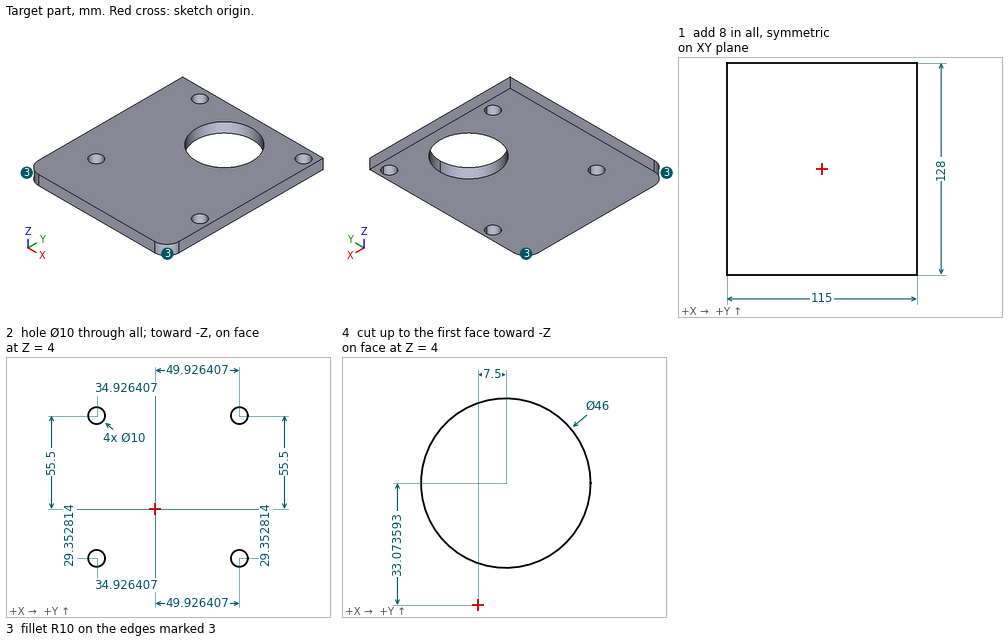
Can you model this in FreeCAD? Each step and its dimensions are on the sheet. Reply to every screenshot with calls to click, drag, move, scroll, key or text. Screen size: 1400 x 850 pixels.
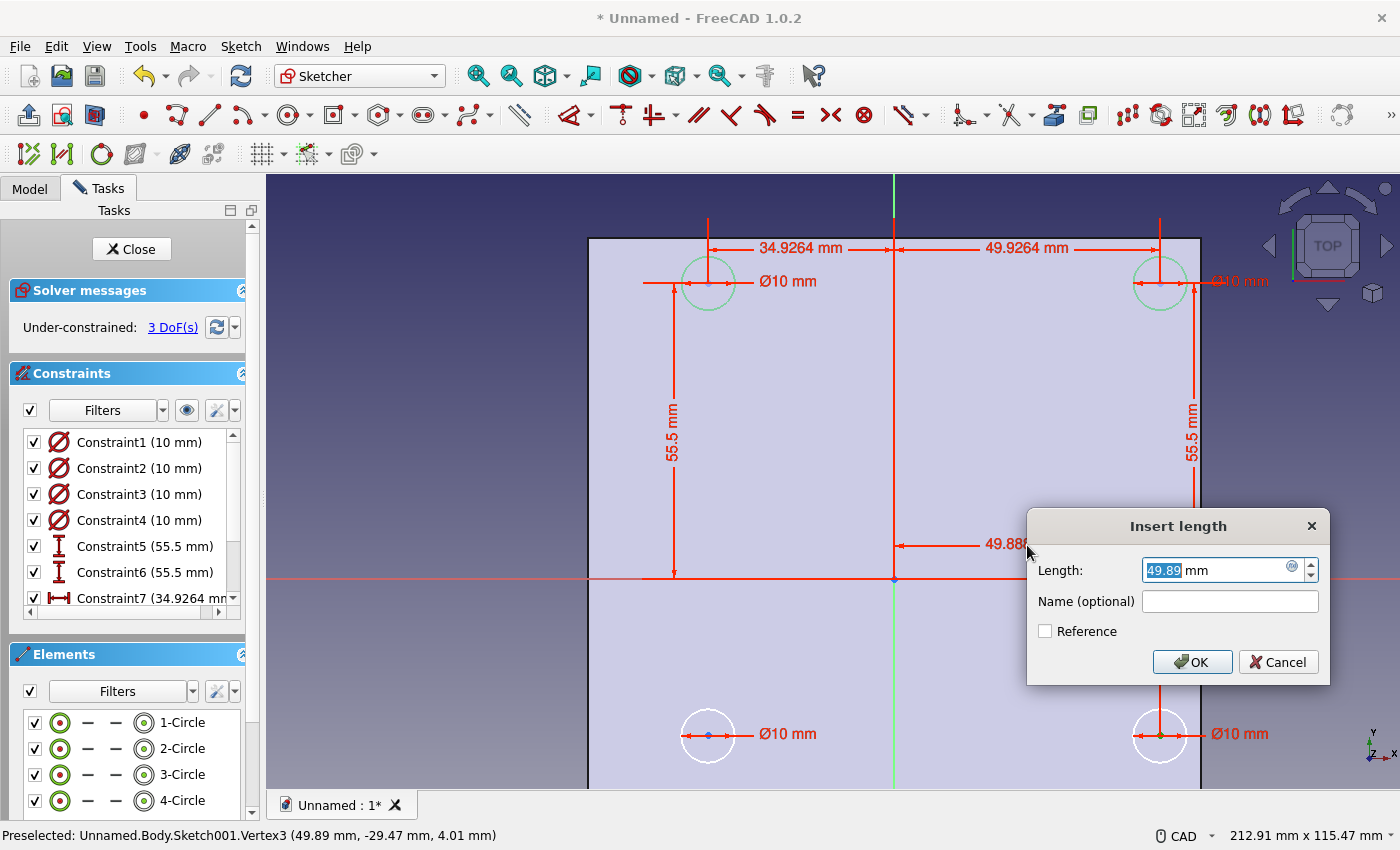
text(49.926407)
key(Return)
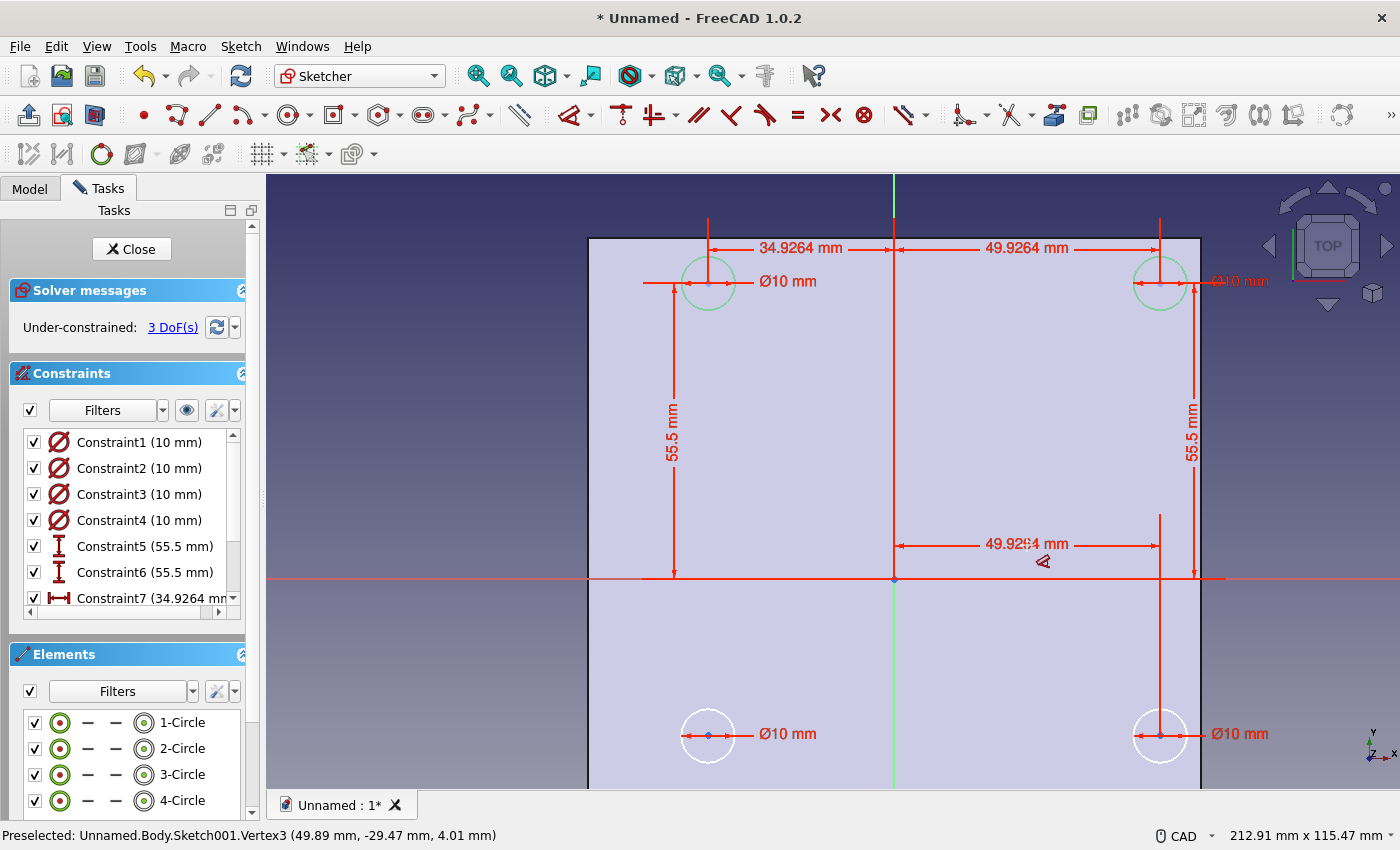
click(1160, 736)
click(1194, 658)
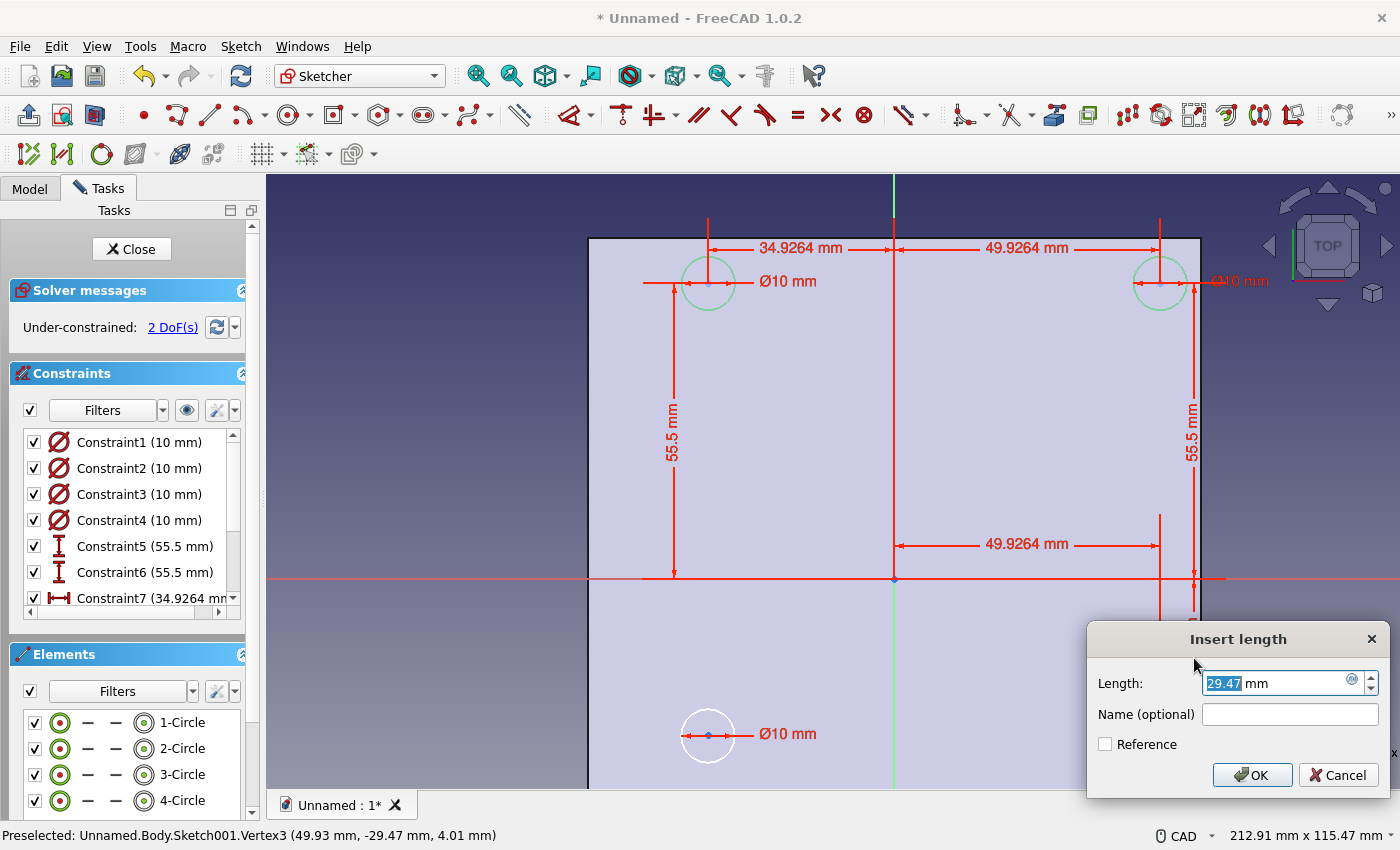
text(29.352814)
key(Return)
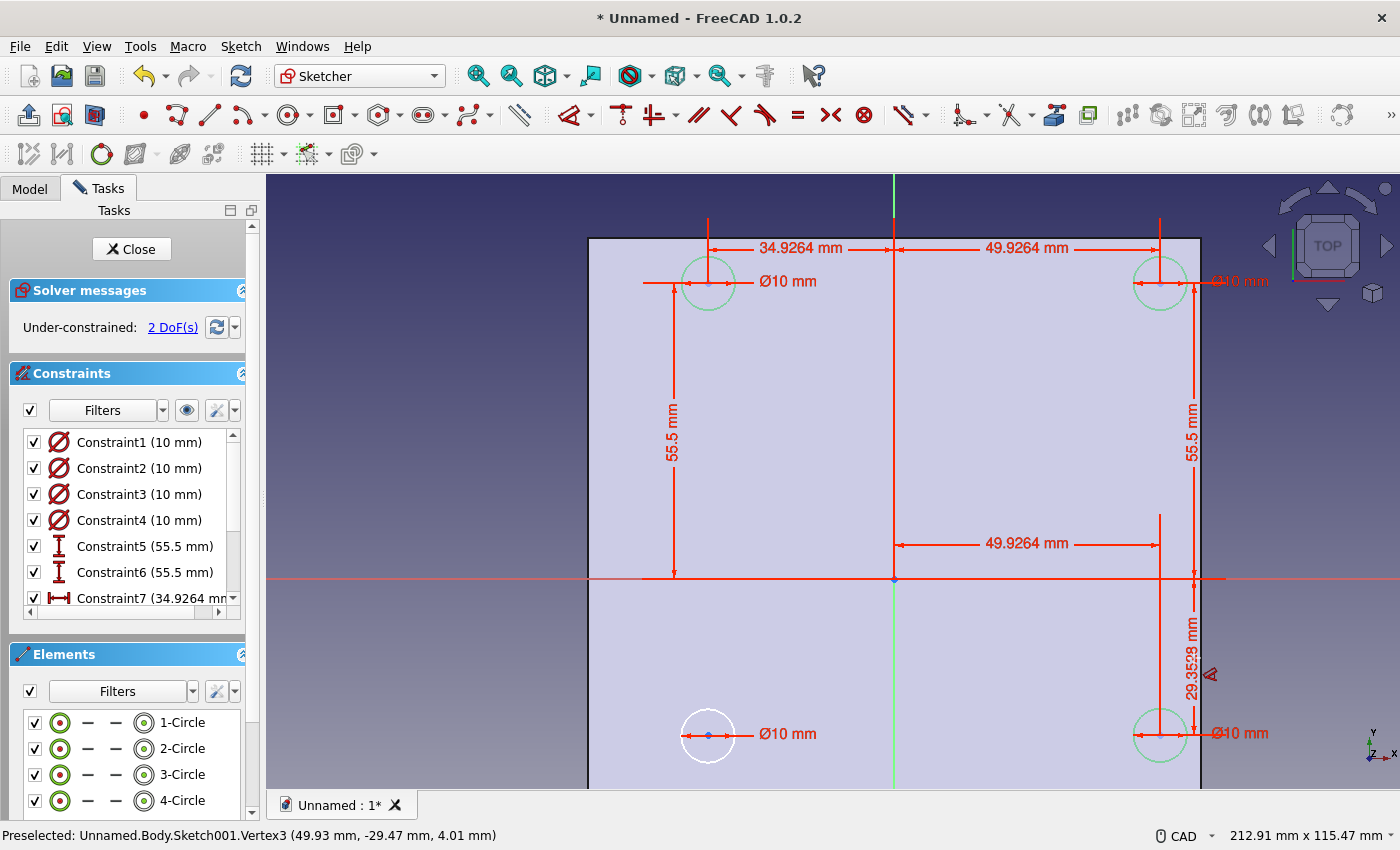
click(708, 736)
click(801, 545)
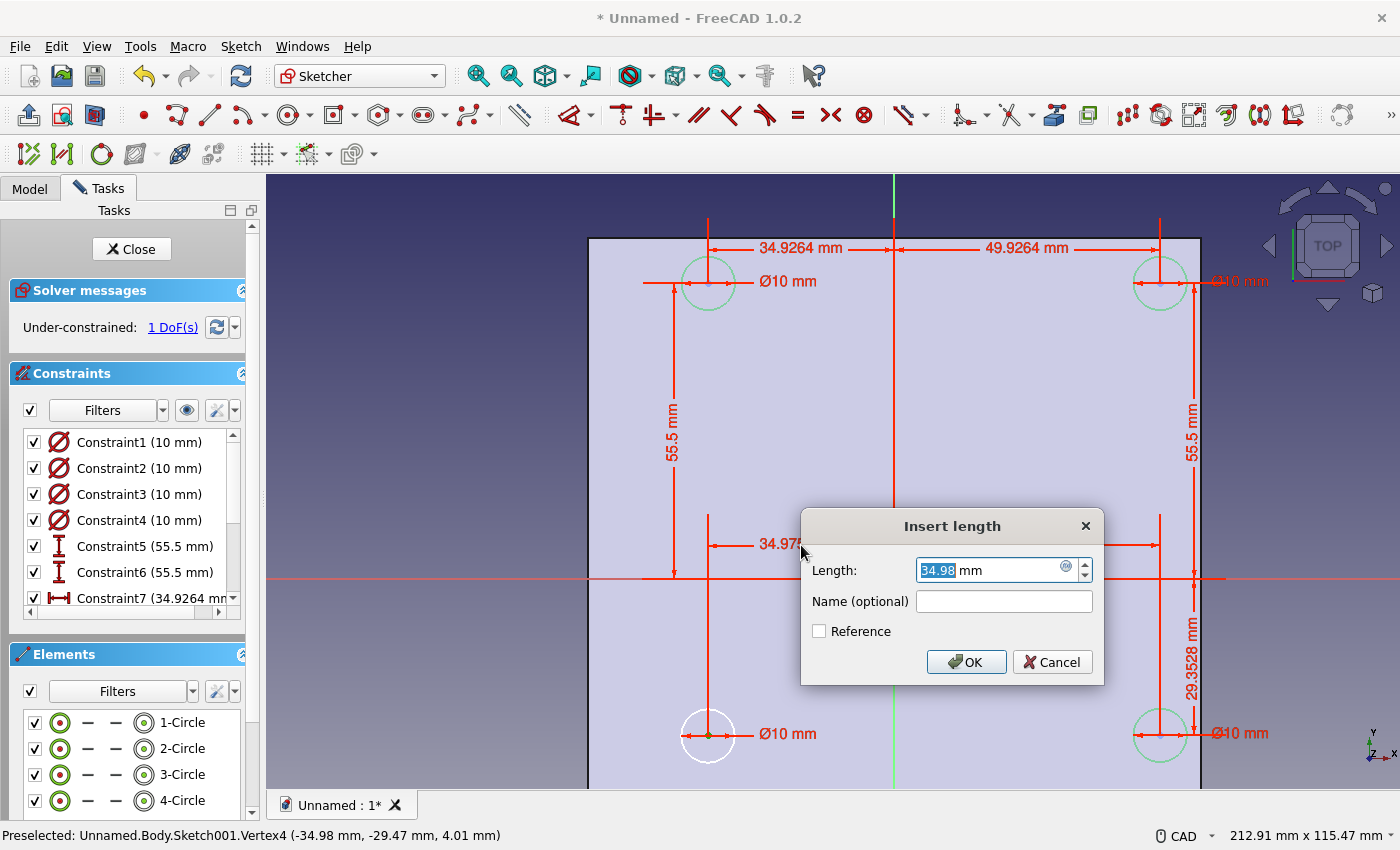
text(34.926407)
key(Return)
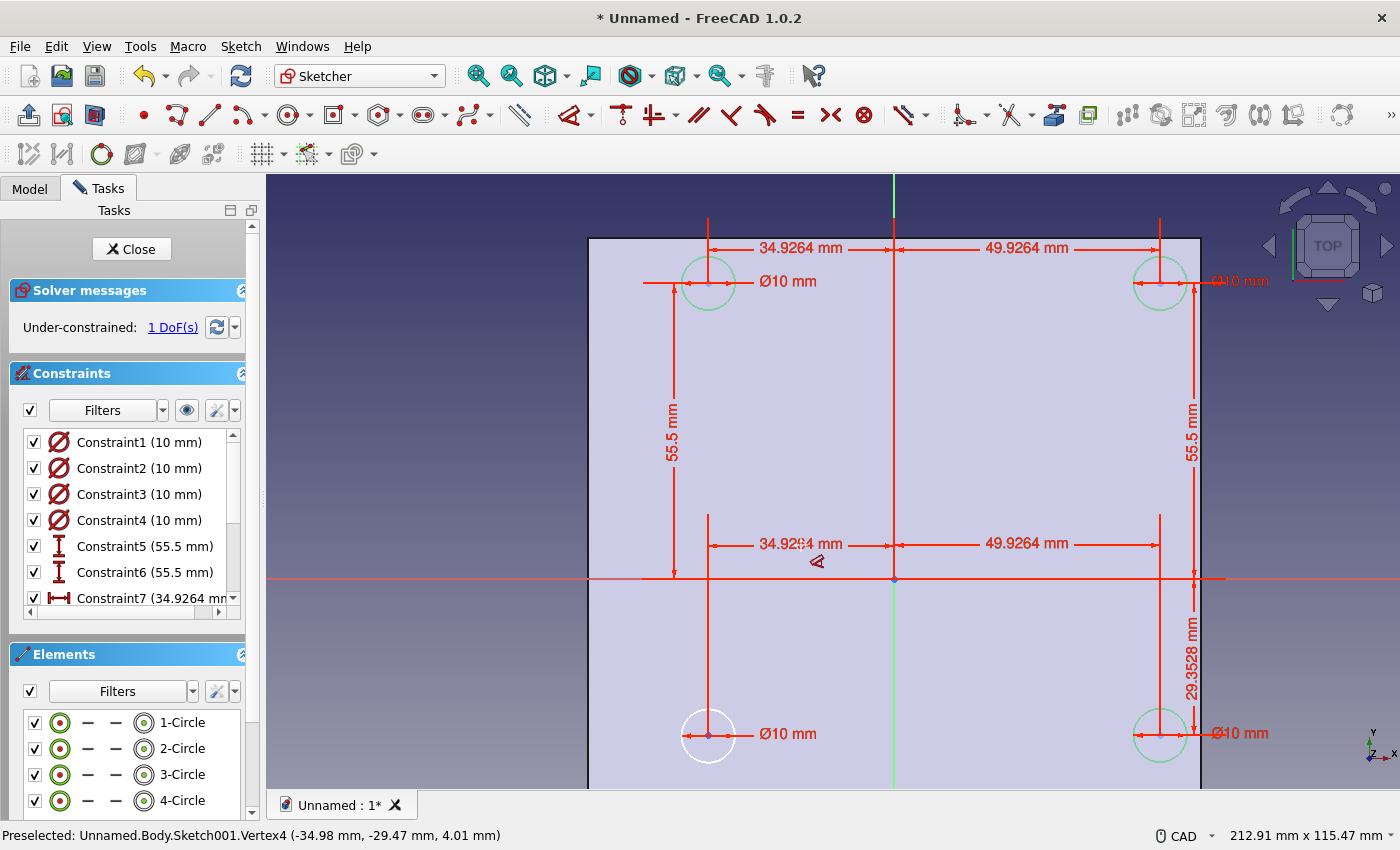
click(708, 736)
click(674, 658)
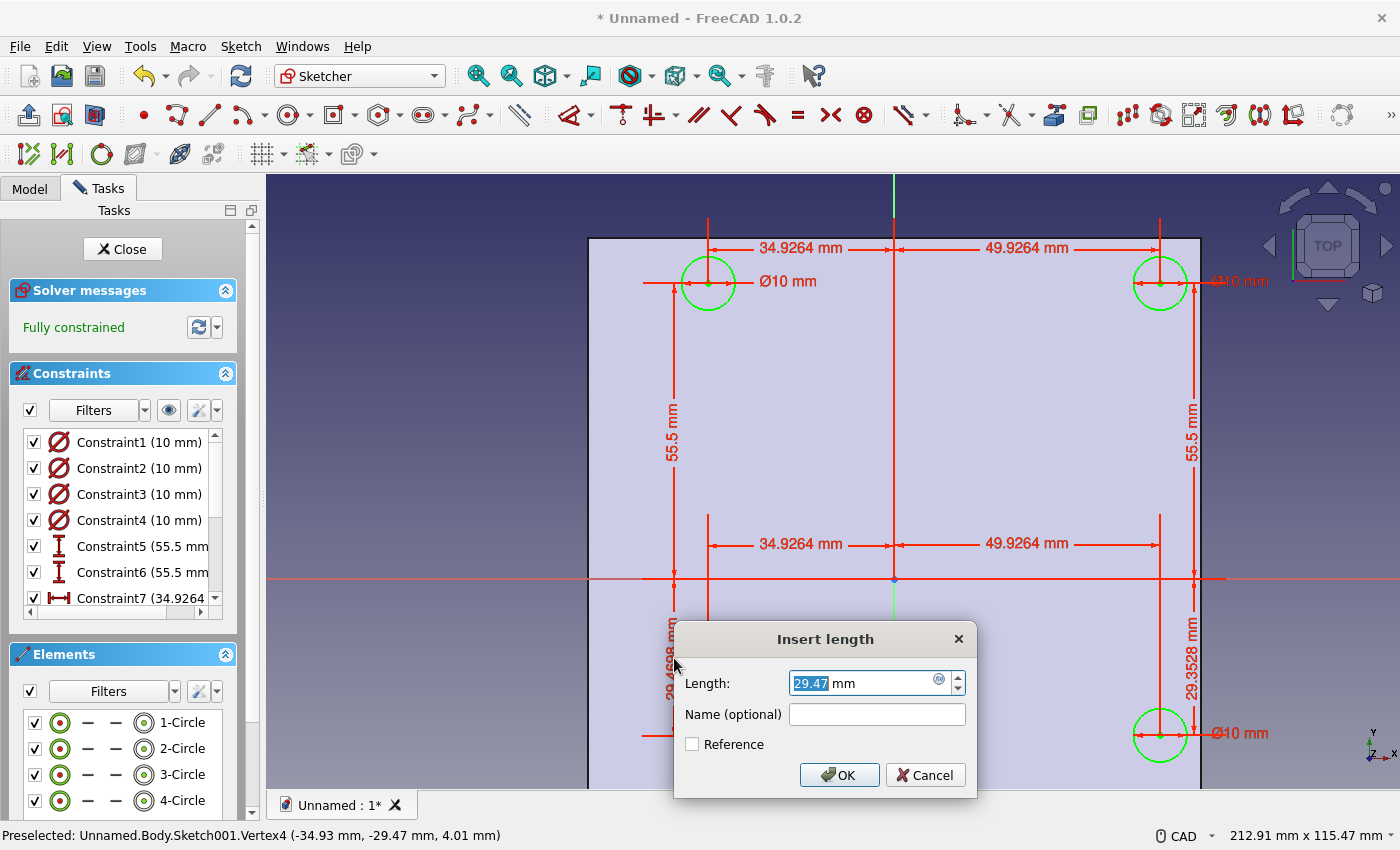
text(29.352814)
key(Return)
key(Escape)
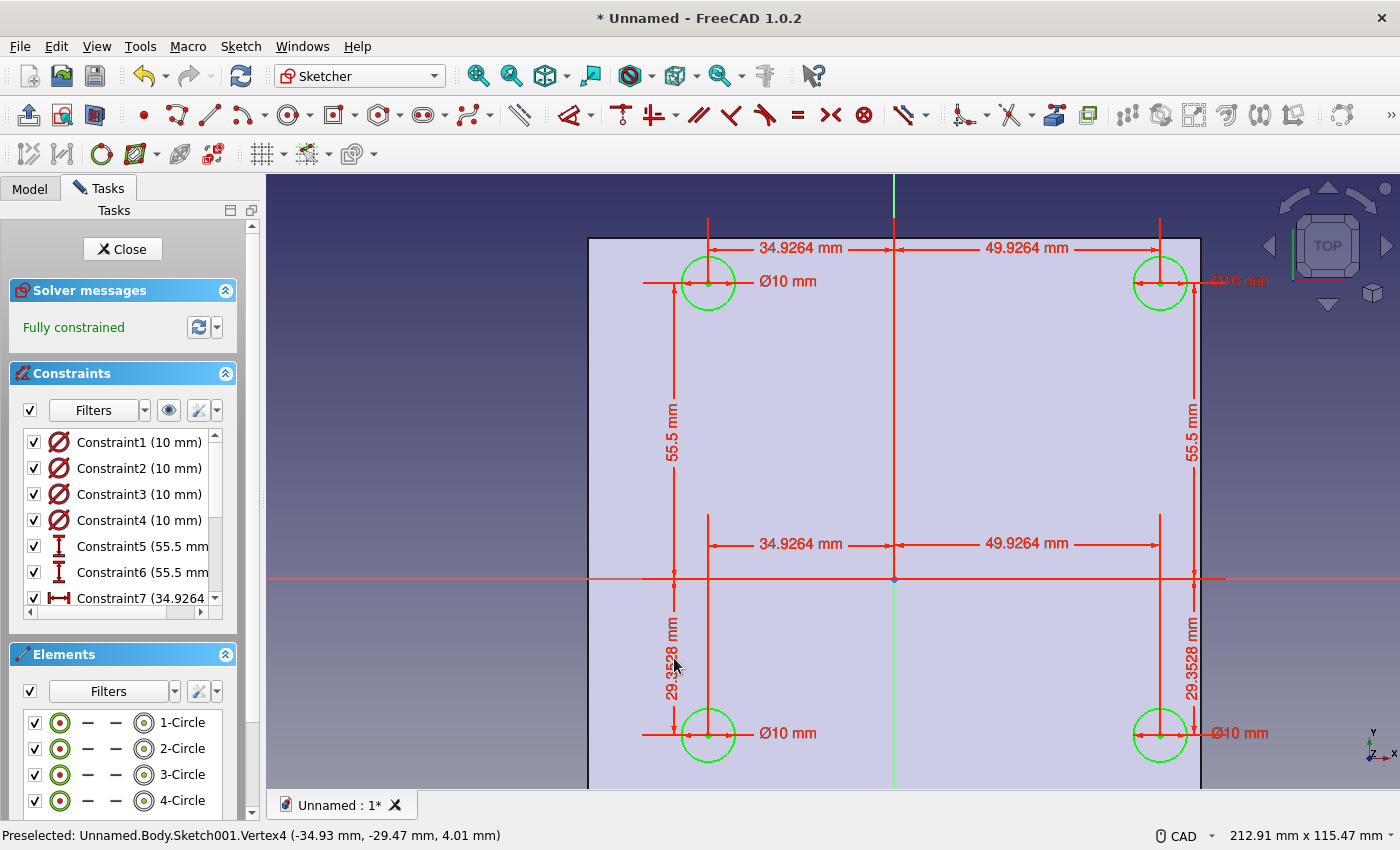
click(123, 249)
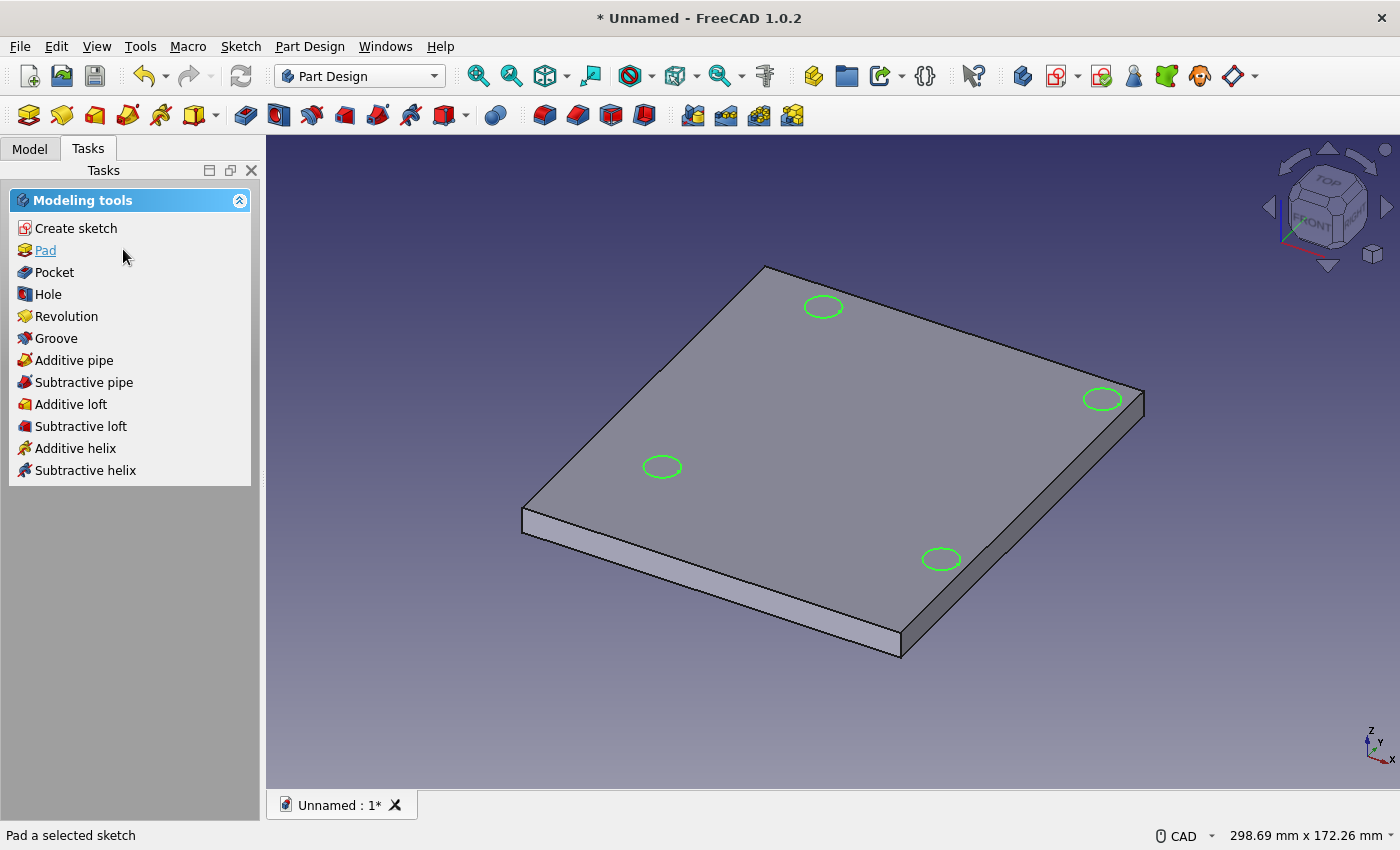
click(279, 116)